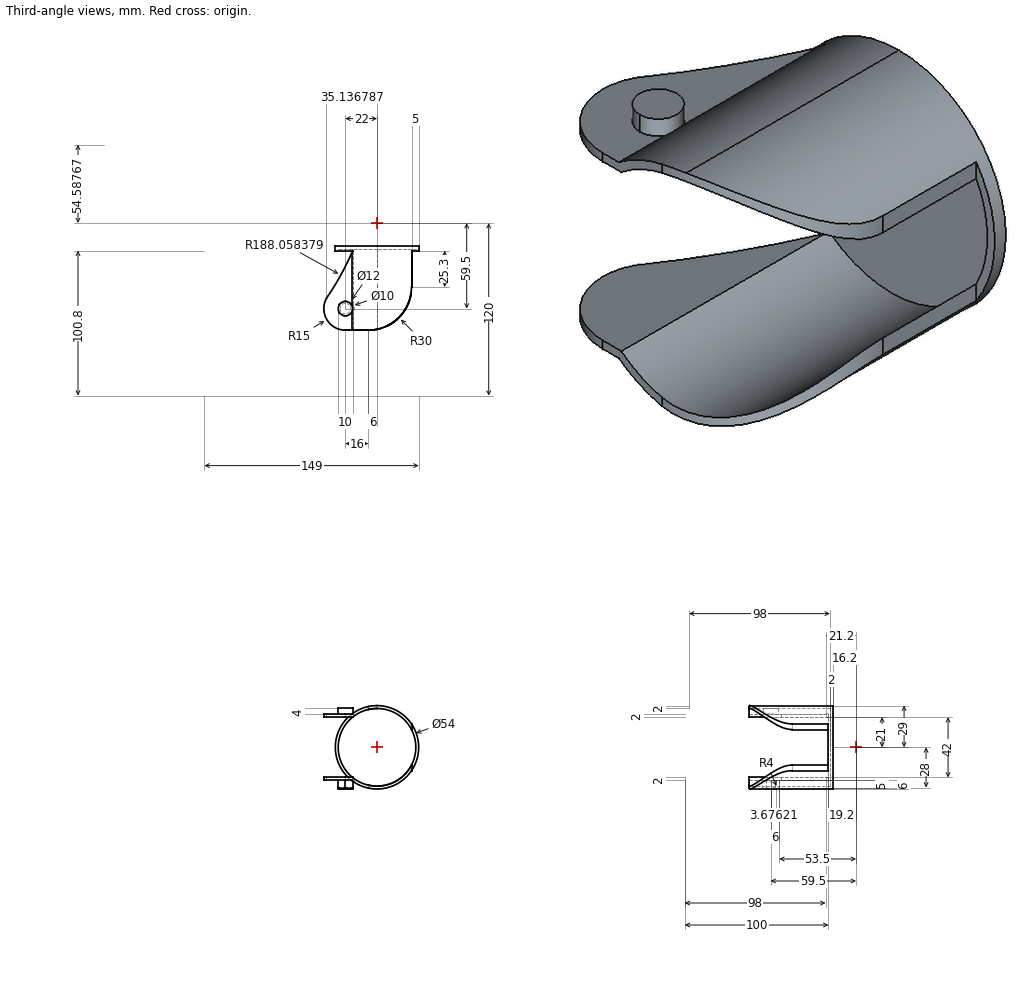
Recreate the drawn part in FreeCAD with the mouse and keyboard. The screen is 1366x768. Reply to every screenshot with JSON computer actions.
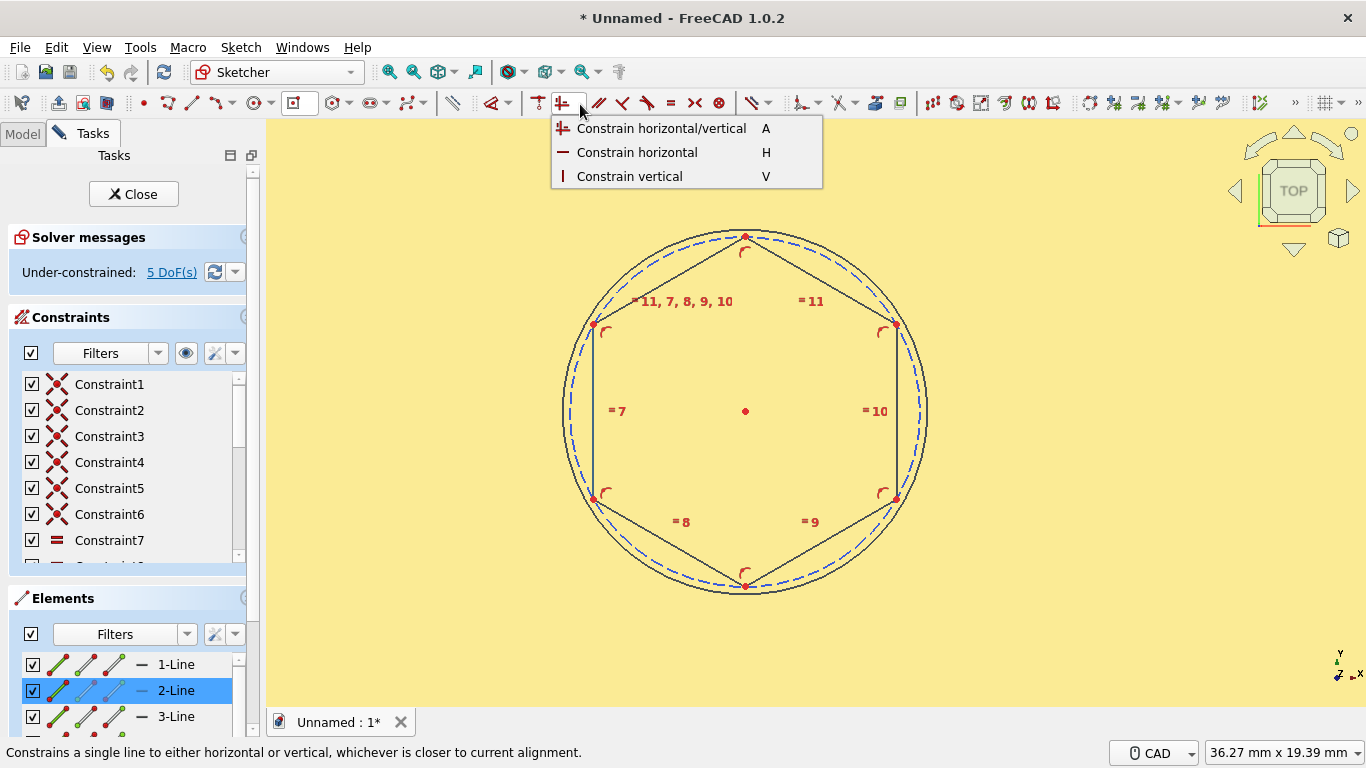
{"action": "left_click", "coordinate": [687, 176]}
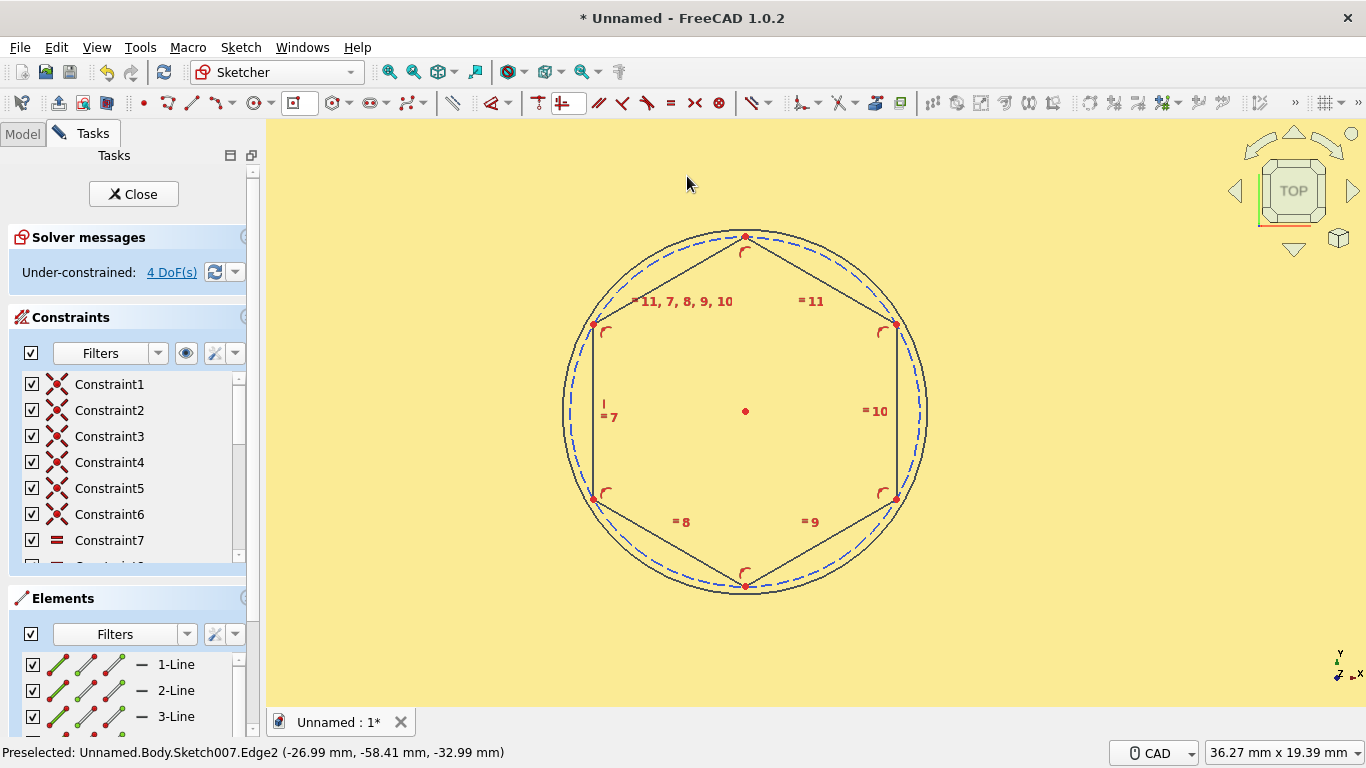
{"action": "key", "text": "d"}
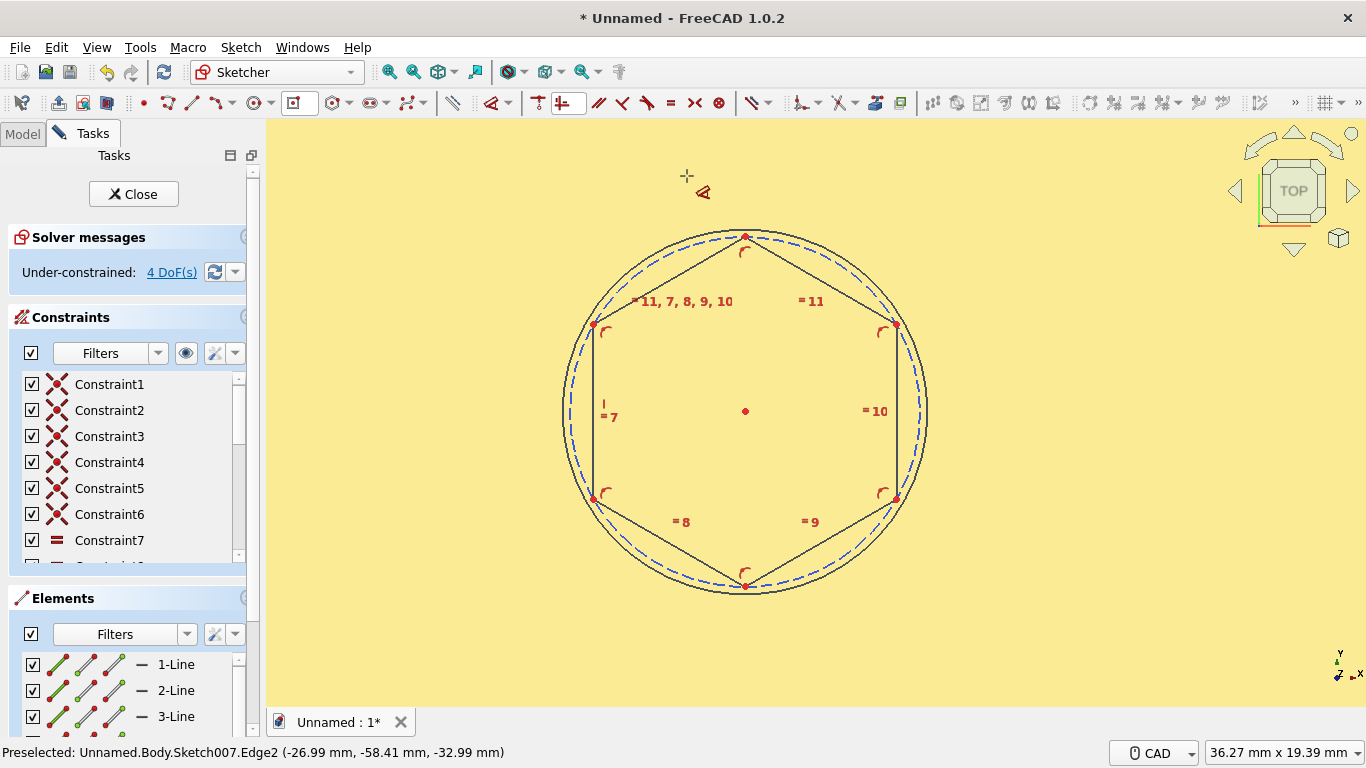
{"action": "scroll", "coordinate": [750, 230], "scroll_direction": "up", "scroll_amount": 4}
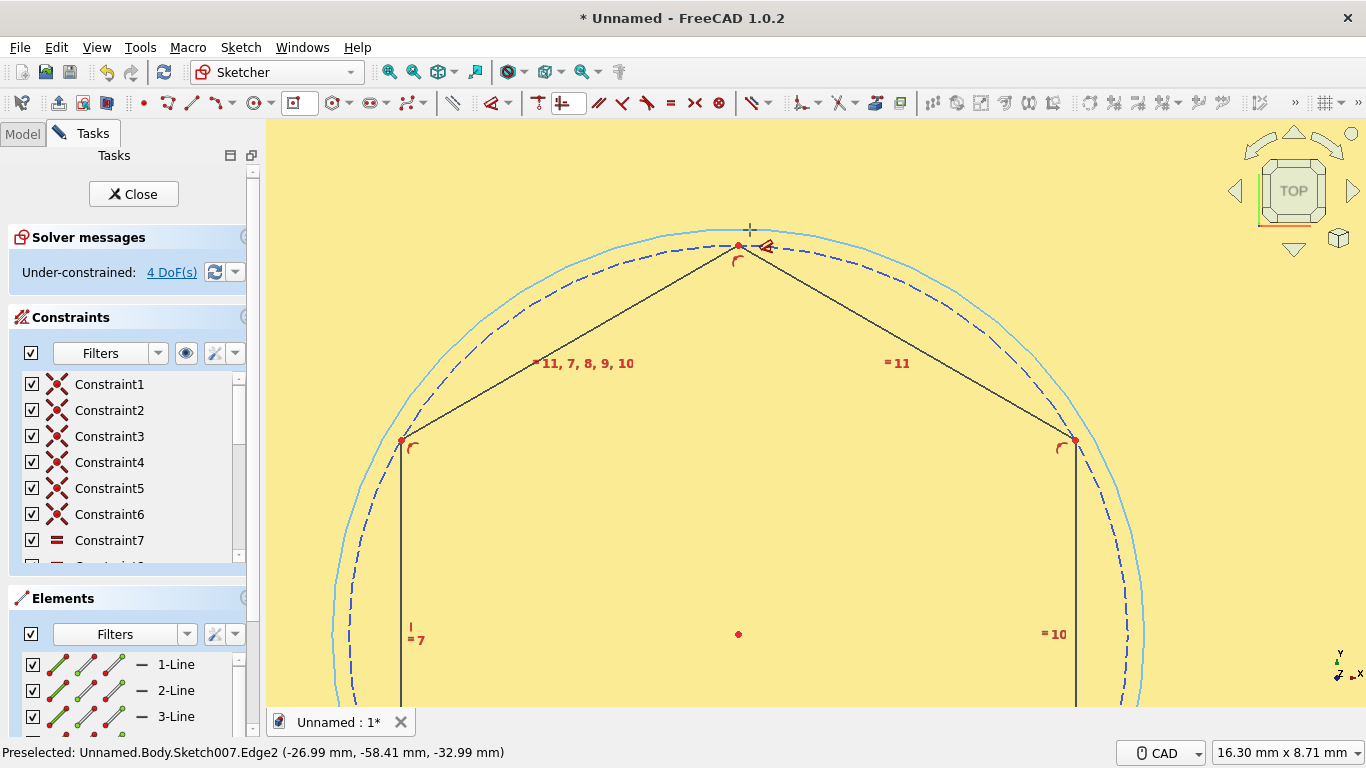
{"action": "left_click", "coordinate": [750, 229]}
{"action": "left_click", "coordinate": [751, 197]}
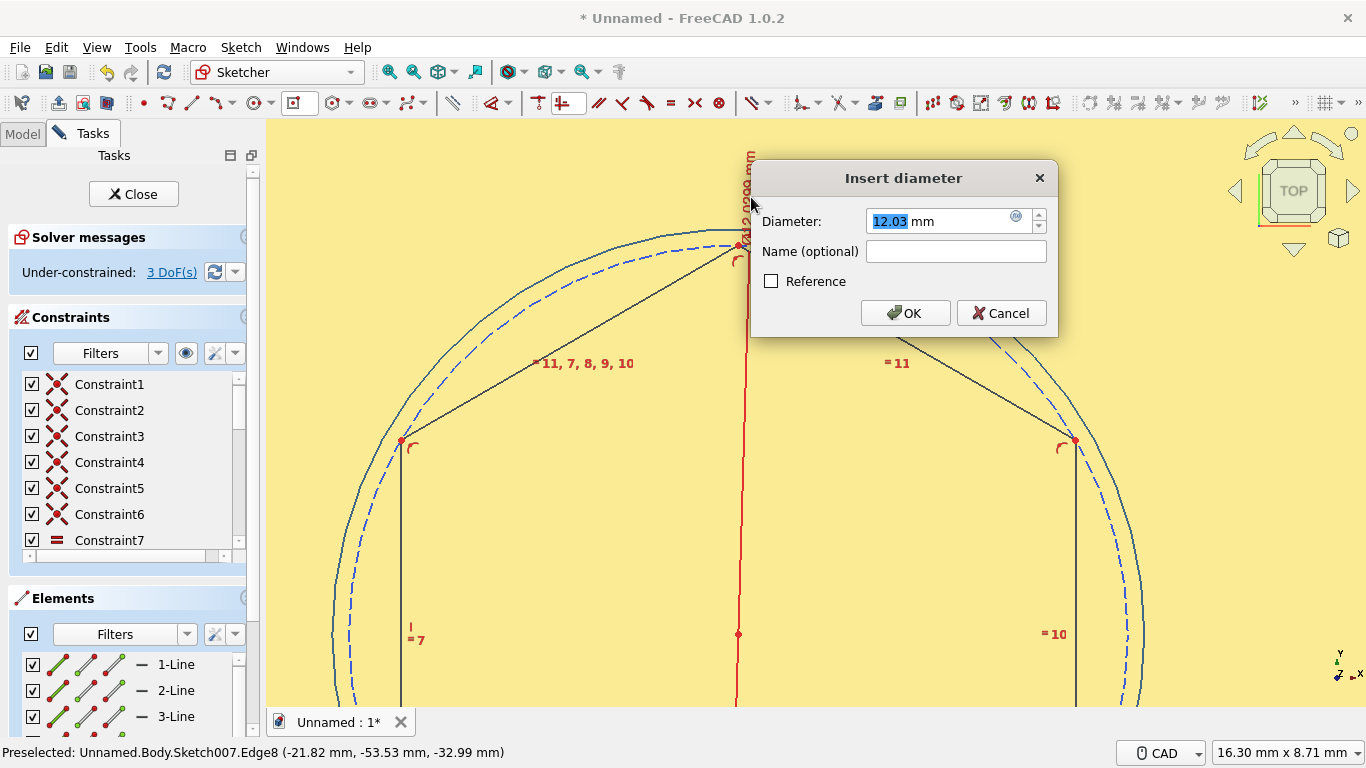
{"action": "type", "text": "12"}
{"action": "key", "text": "Return"}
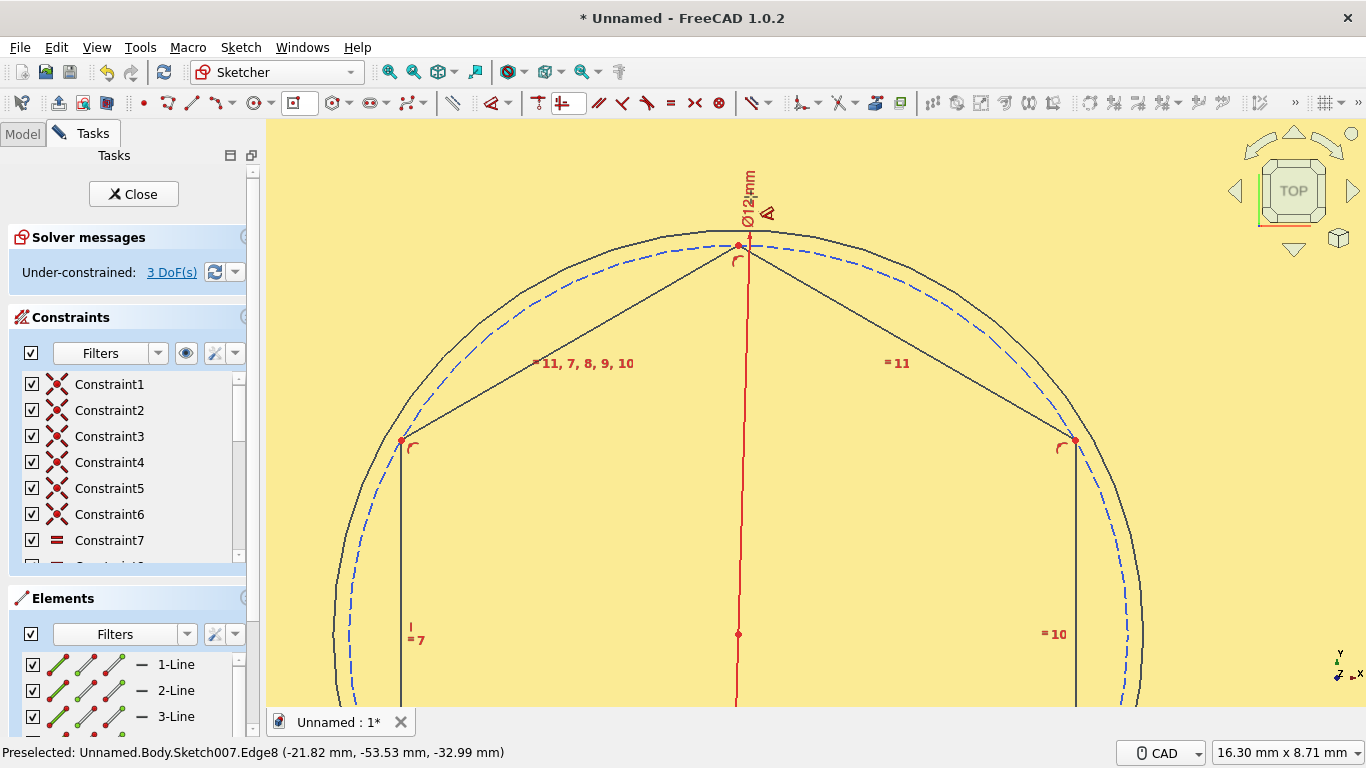
{"action": "left_click", "coordinate": [401, 440]}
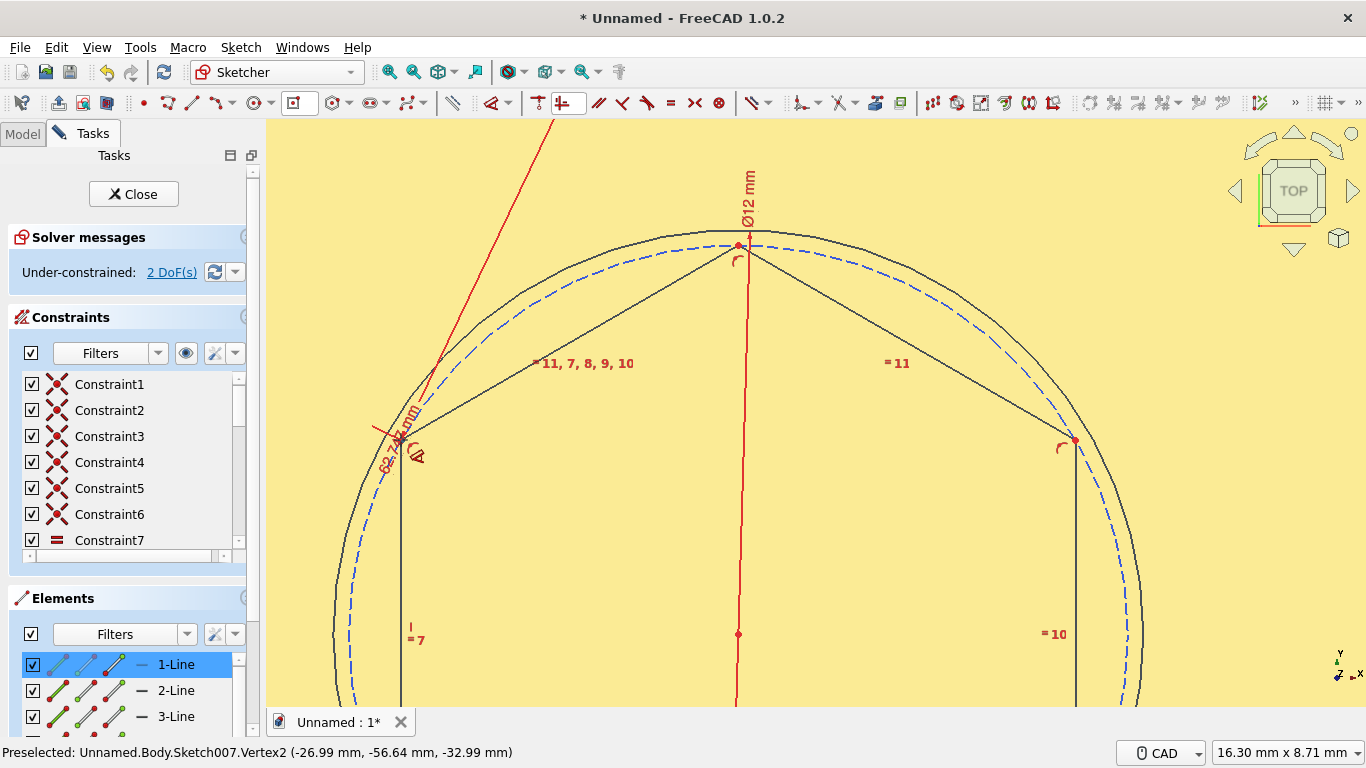
{"action": "scroll", "coordinate": [755, 234], "scroll_direction": "down", "scroll_amount": 4}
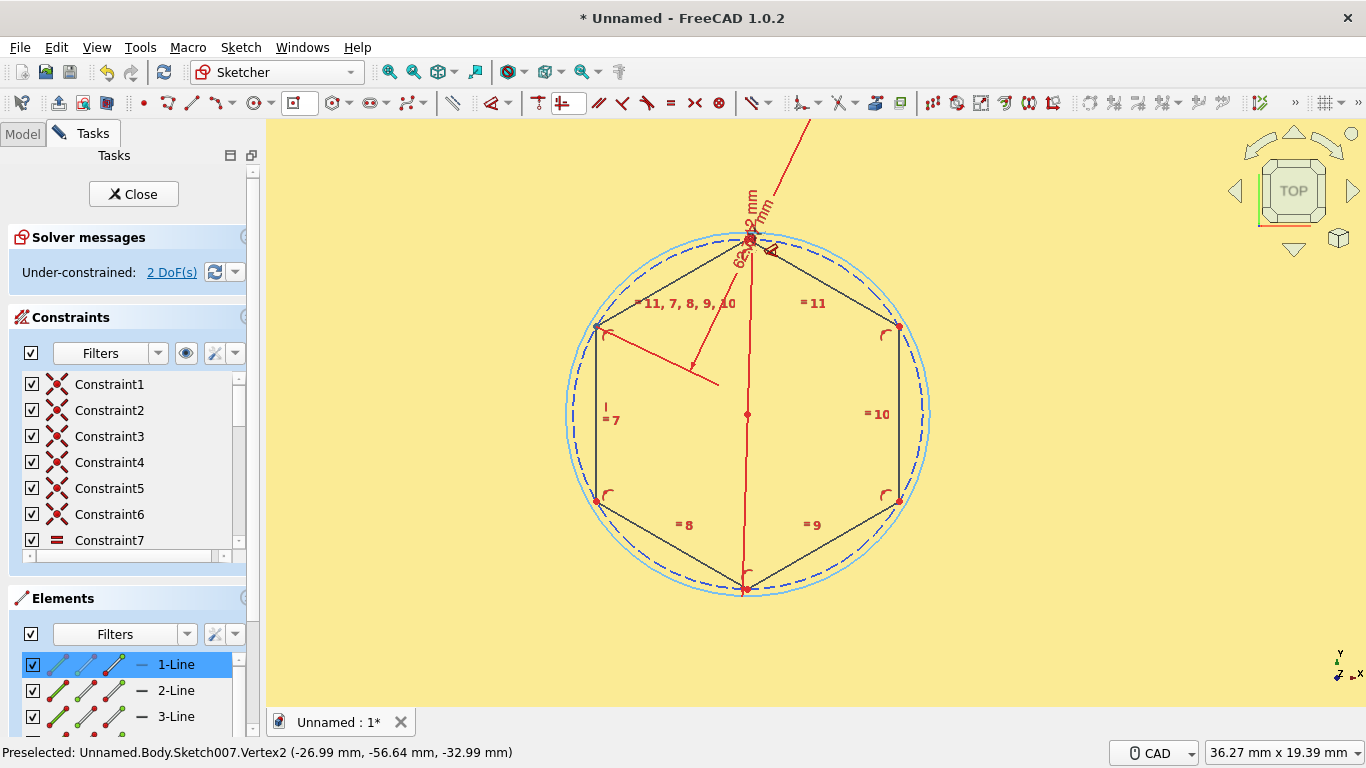
{"action": "left_click", "coordinate": [899, 502]}
{"action": "left_click", "coordinate": [748, 536]}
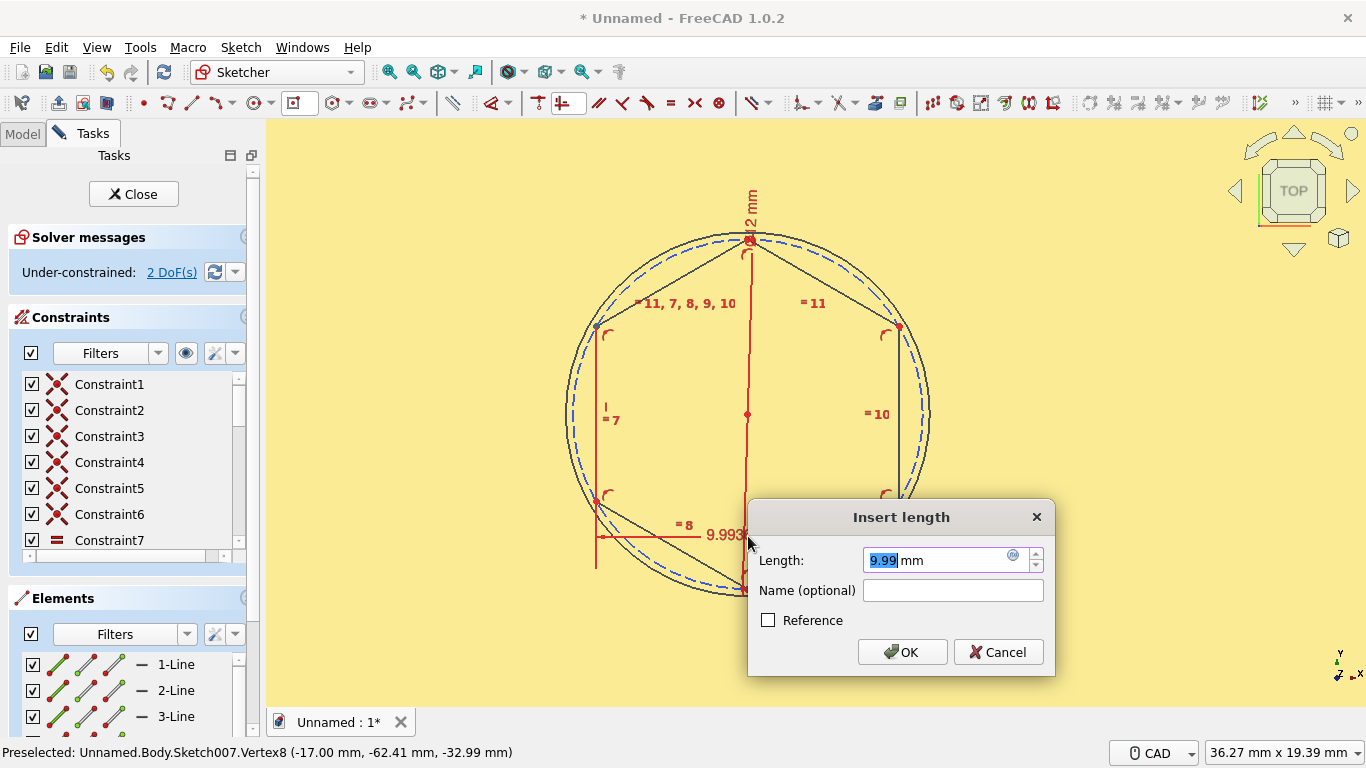
{"action": "type", "text": "10"}
{"action": "key", "text": "Return"}